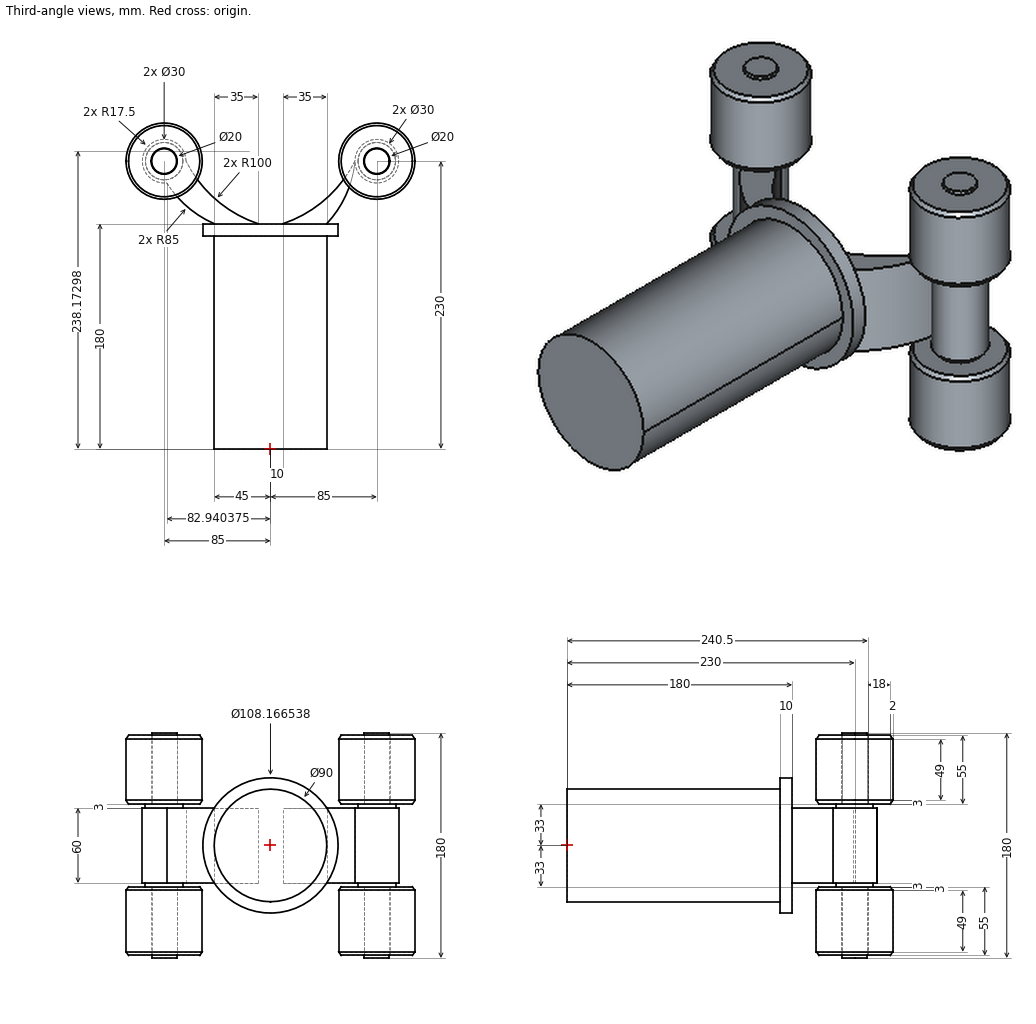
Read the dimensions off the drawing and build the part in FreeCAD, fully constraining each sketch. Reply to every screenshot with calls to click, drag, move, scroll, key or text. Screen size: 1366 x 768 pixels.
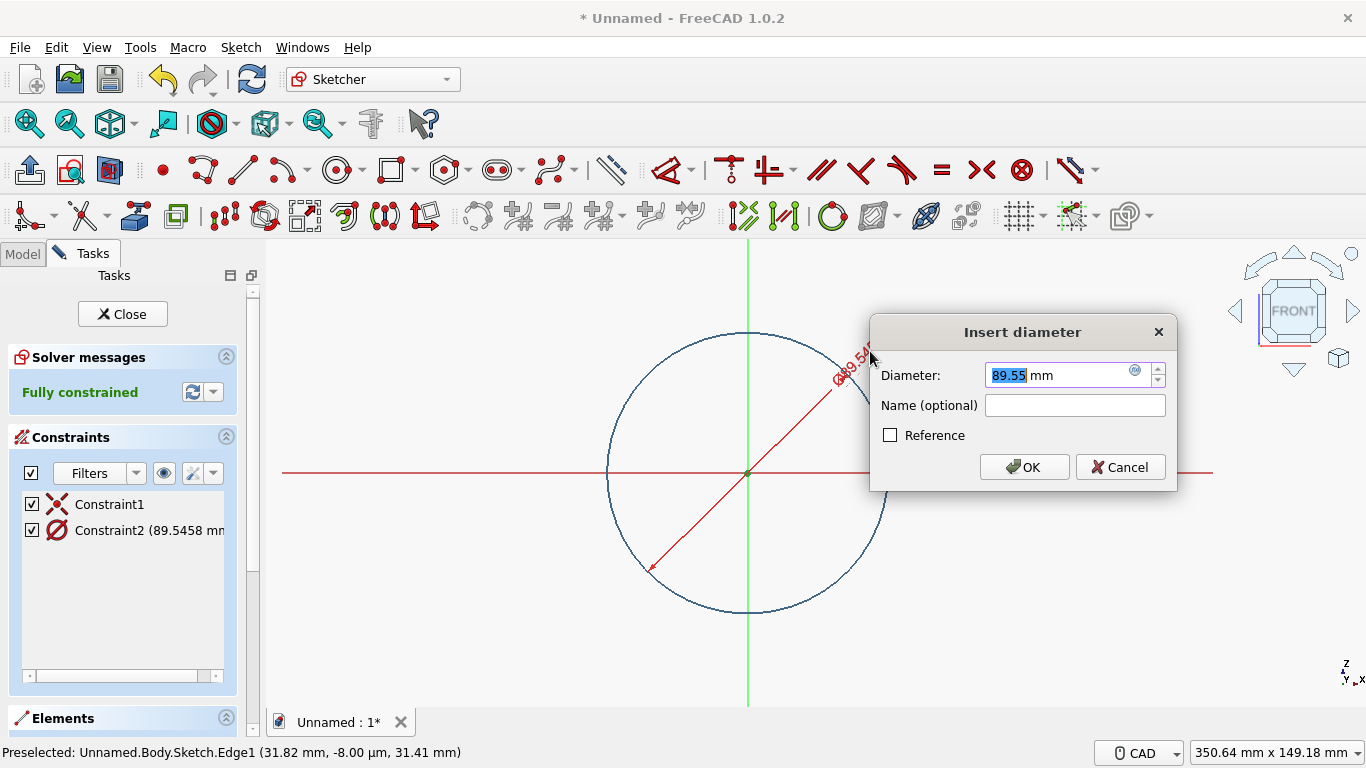
text(90)
key(Return)
key(Escape)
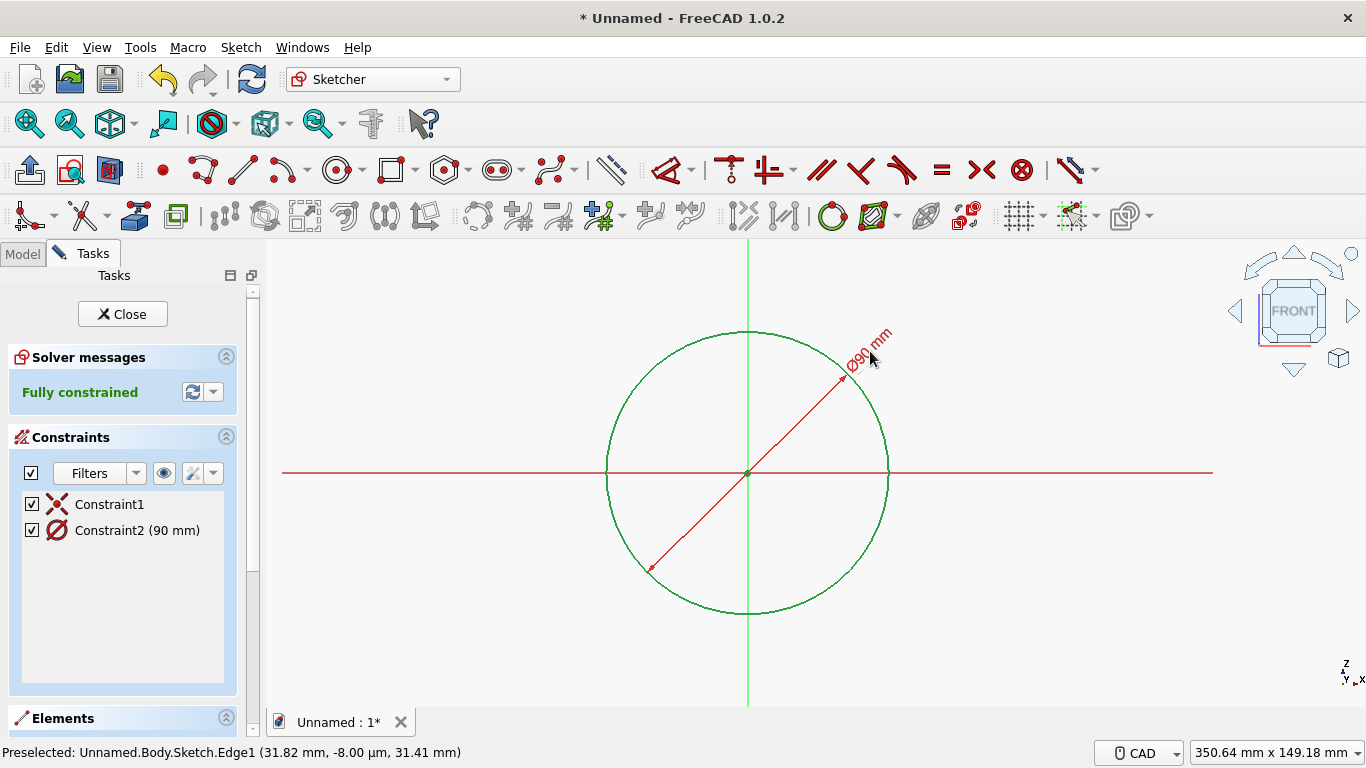
click(123, 314)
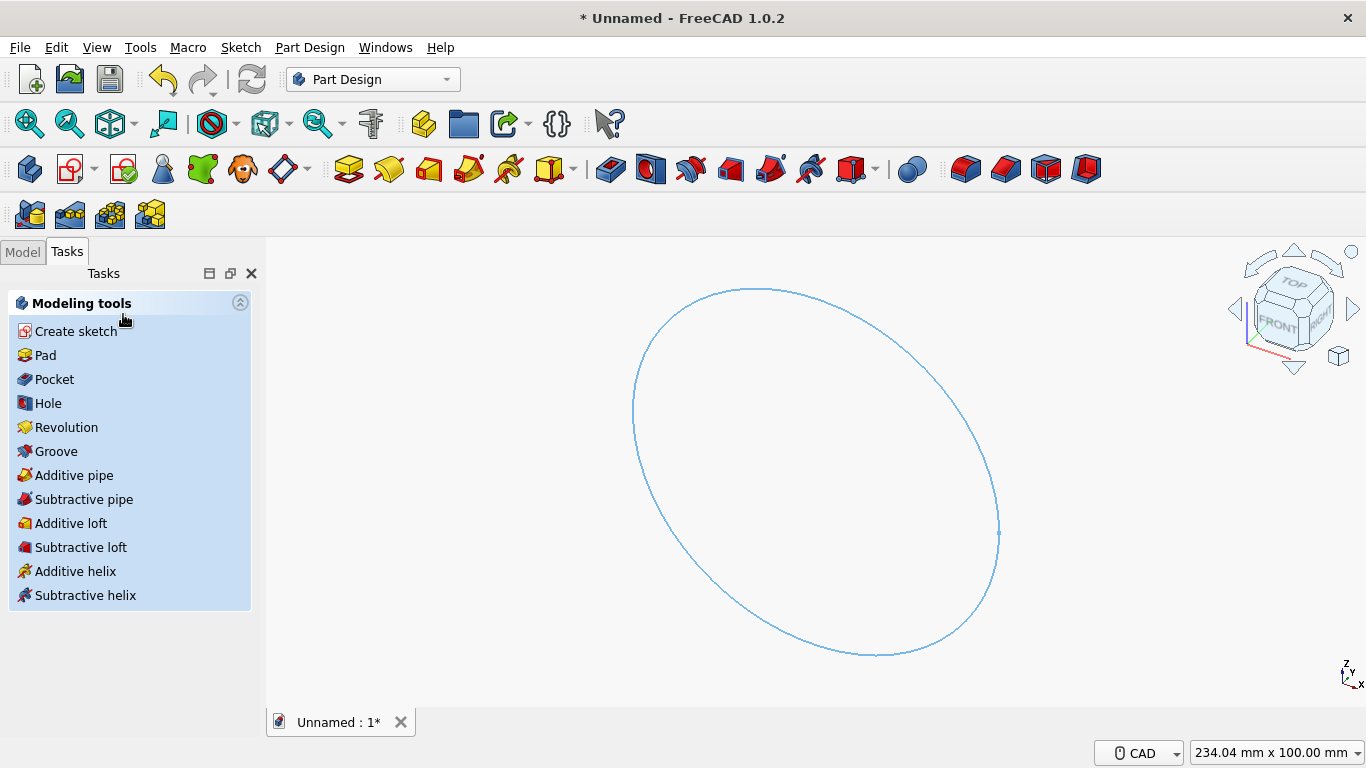
click(350, 170)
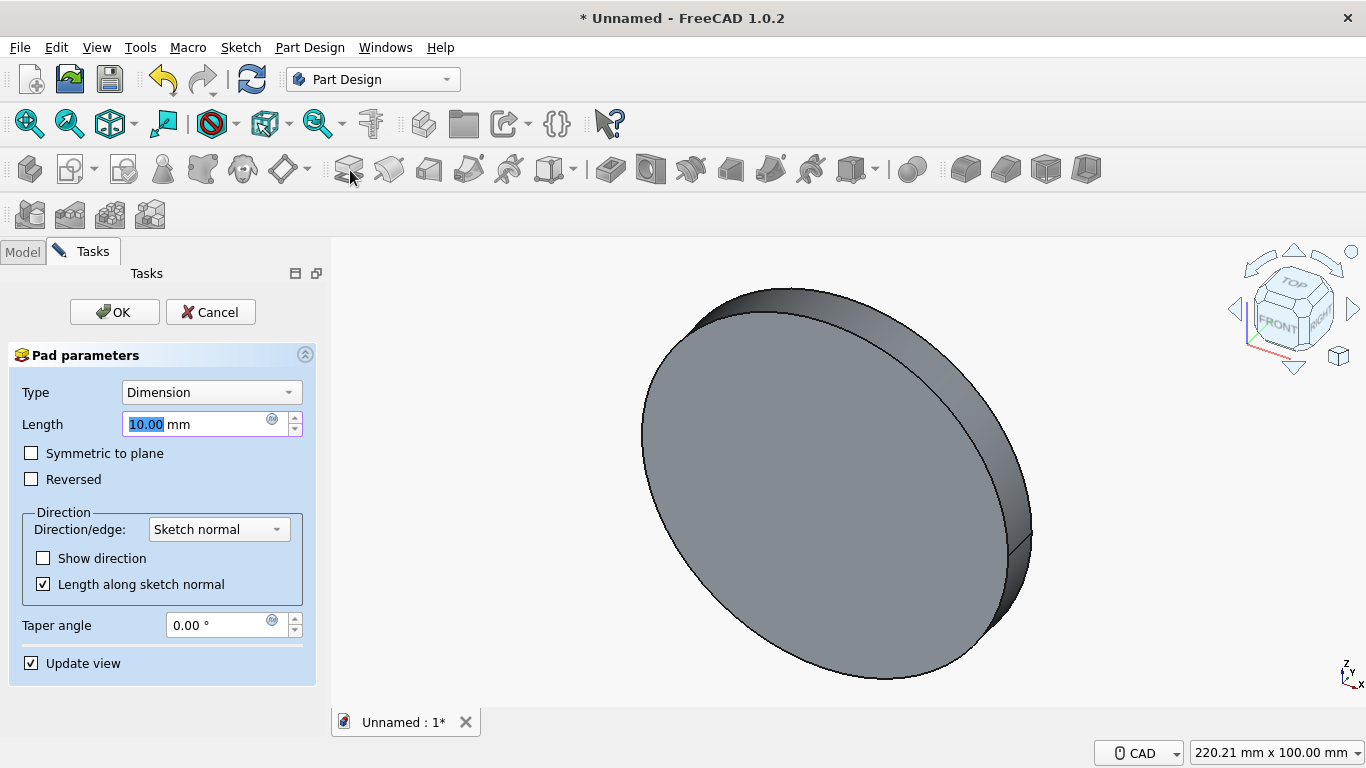
text(180)
key(Tab)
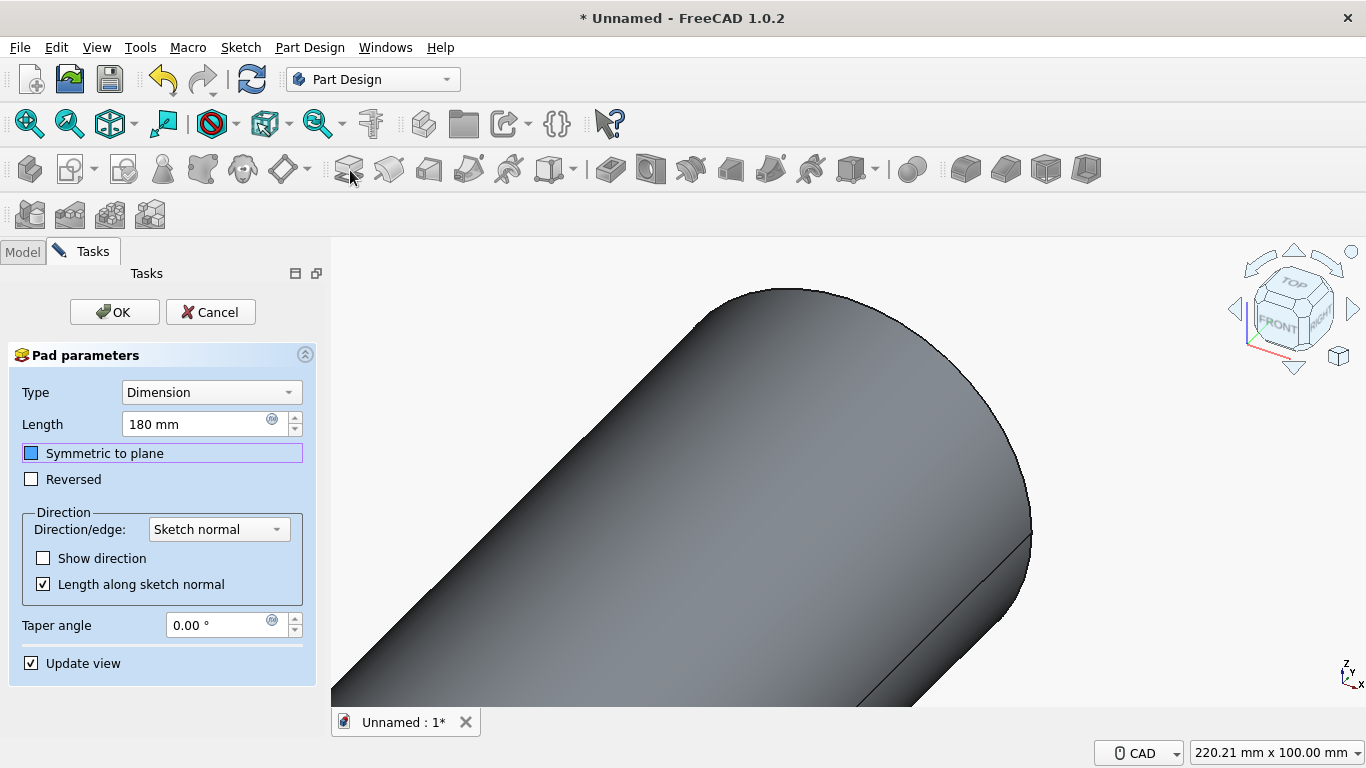
click(30, 479)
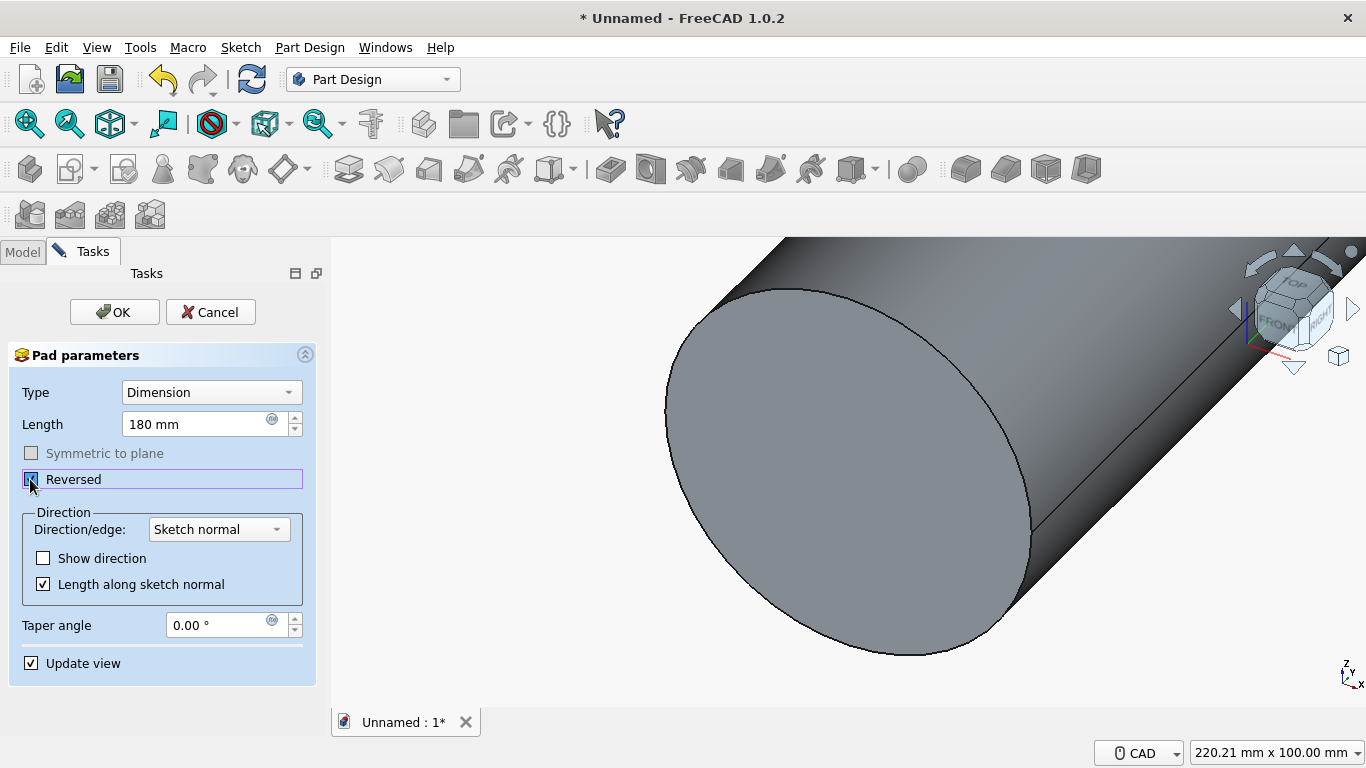
click(115, 312)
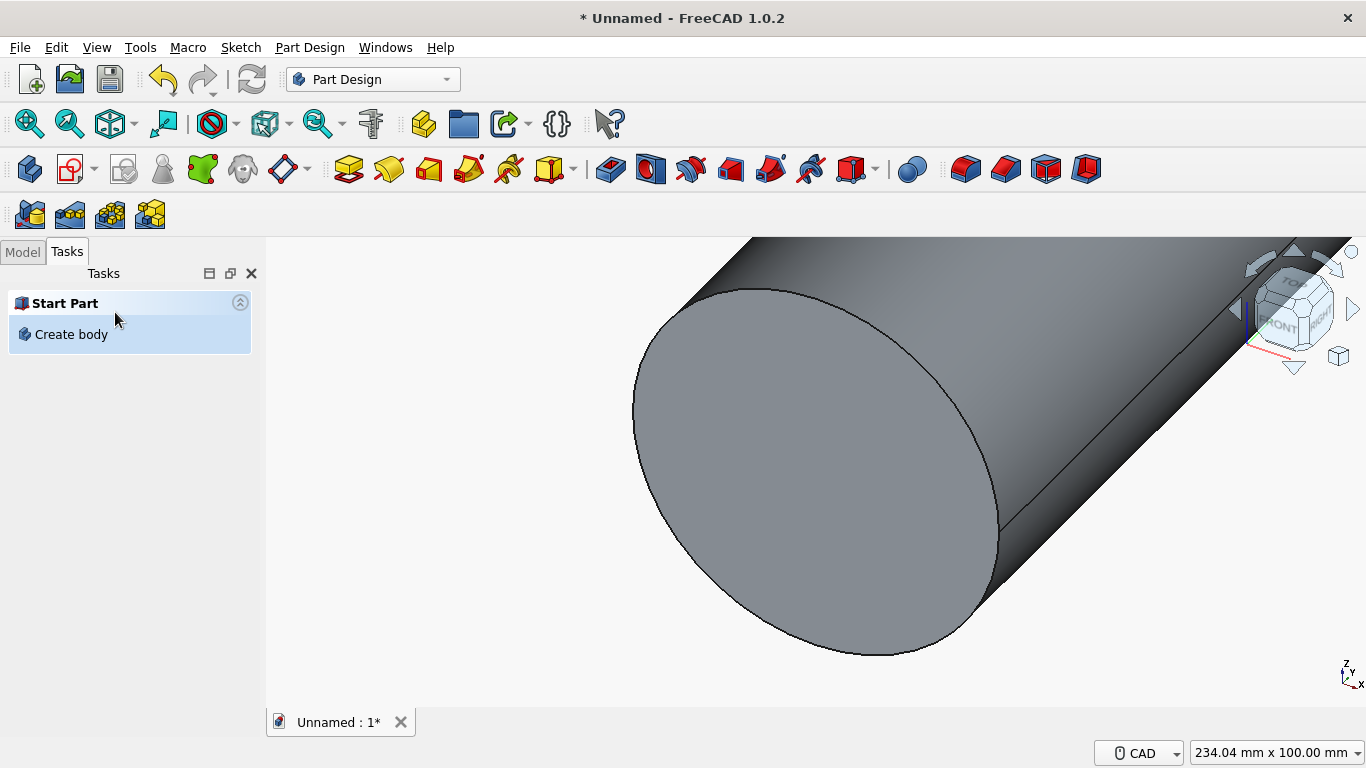
click(30, 124)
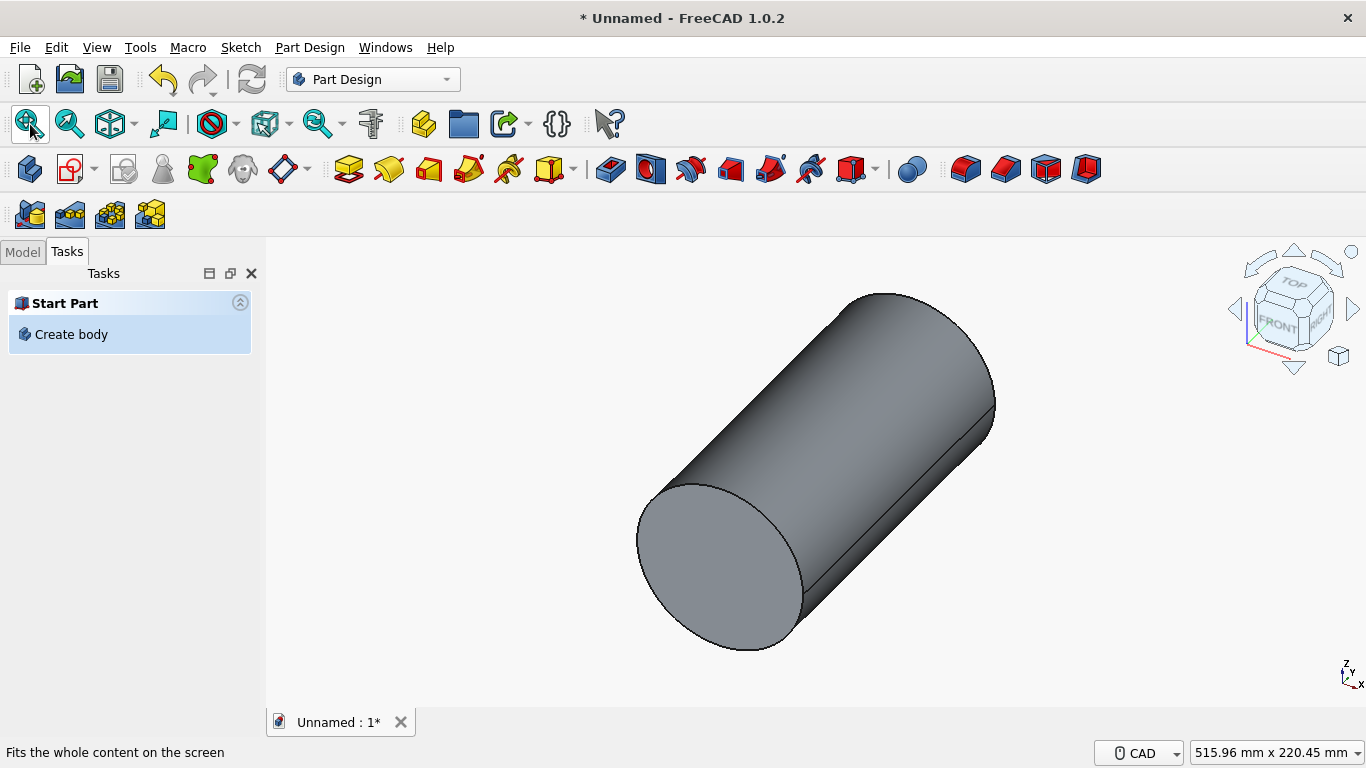
click(30, 170)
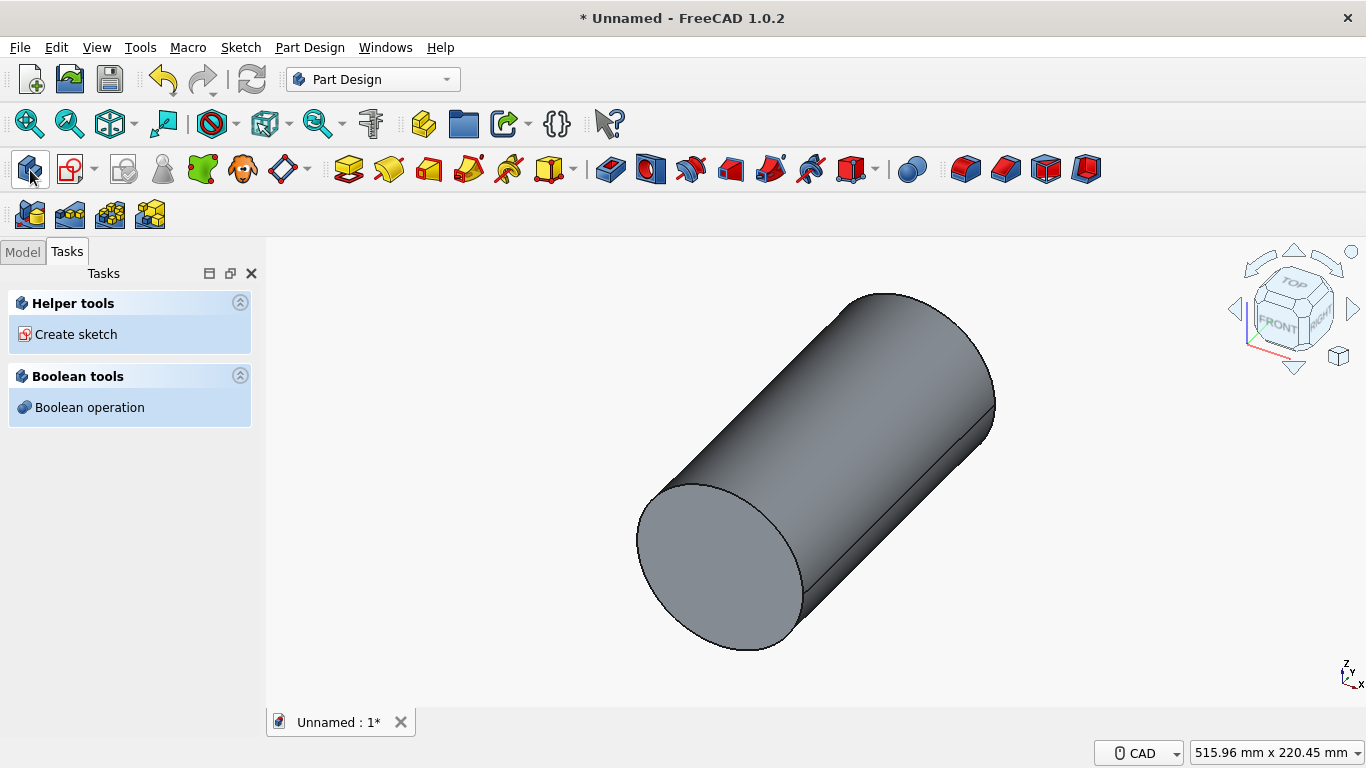
click(306, 667)